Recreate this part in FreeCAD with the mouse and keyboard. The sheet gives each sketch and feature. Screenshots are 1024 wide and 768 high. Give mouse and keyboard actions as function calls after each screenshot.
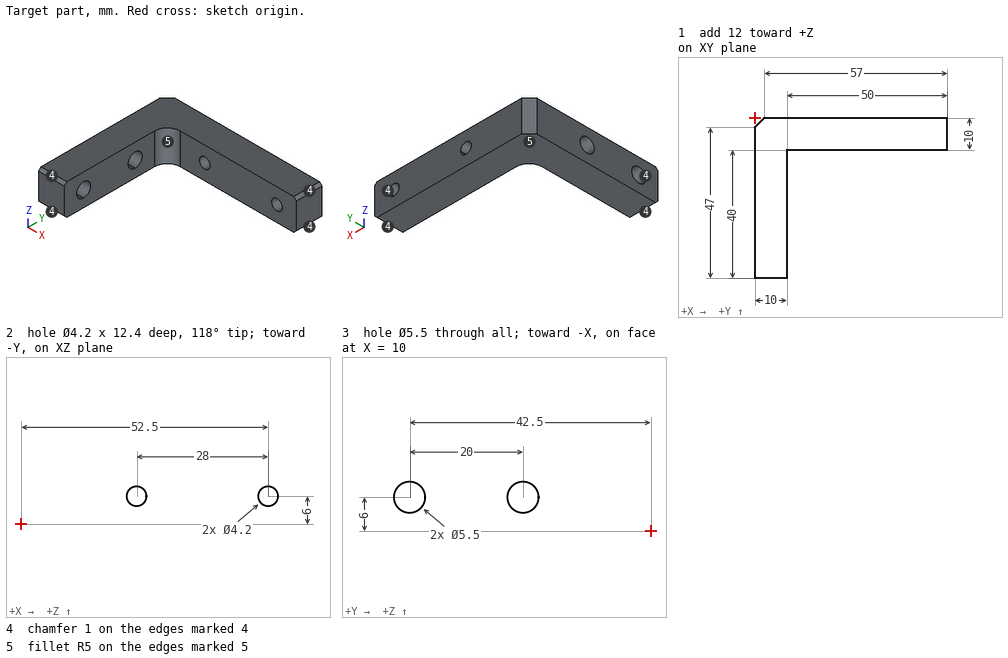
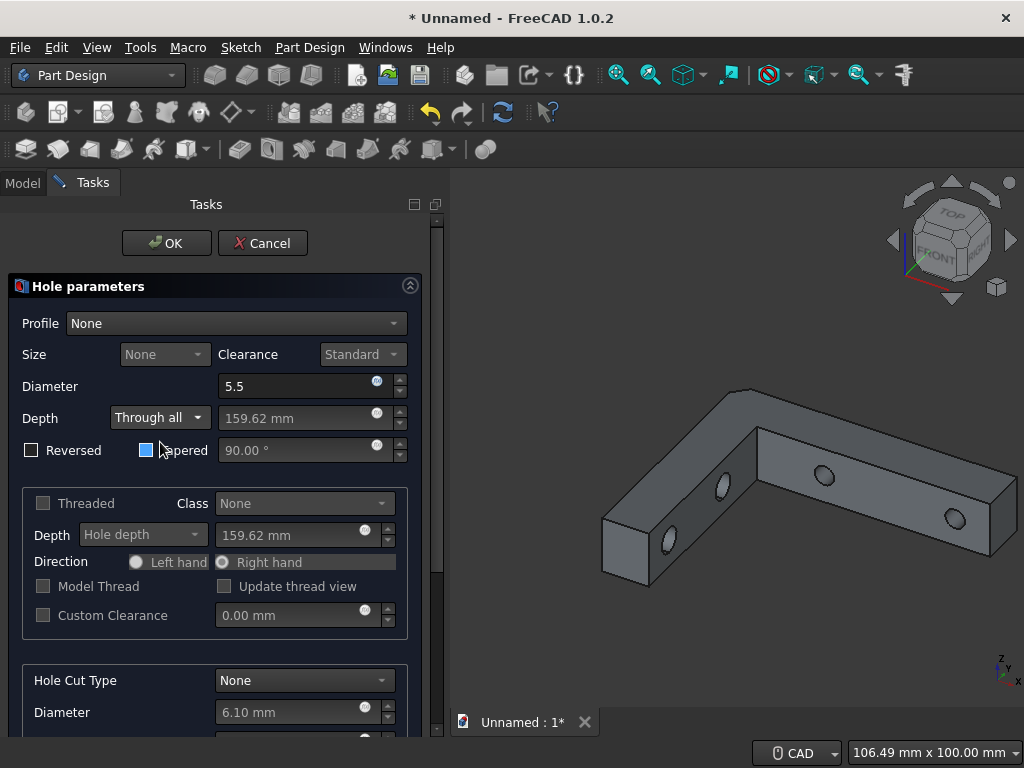
click(167, 243)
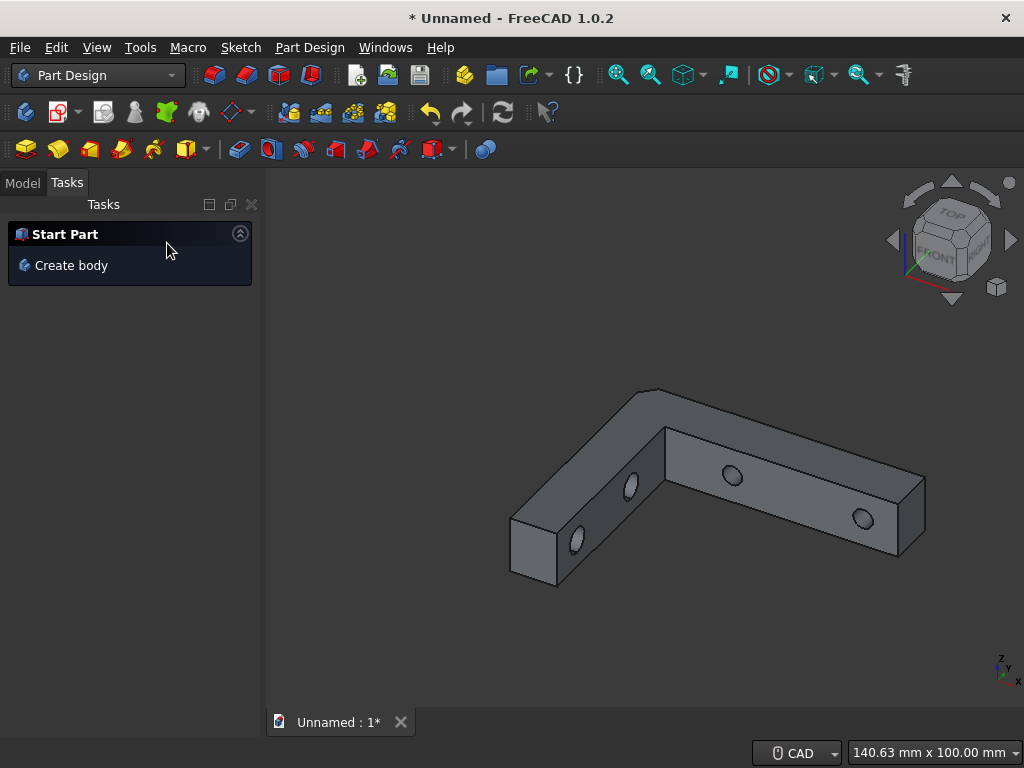
click(534, 525)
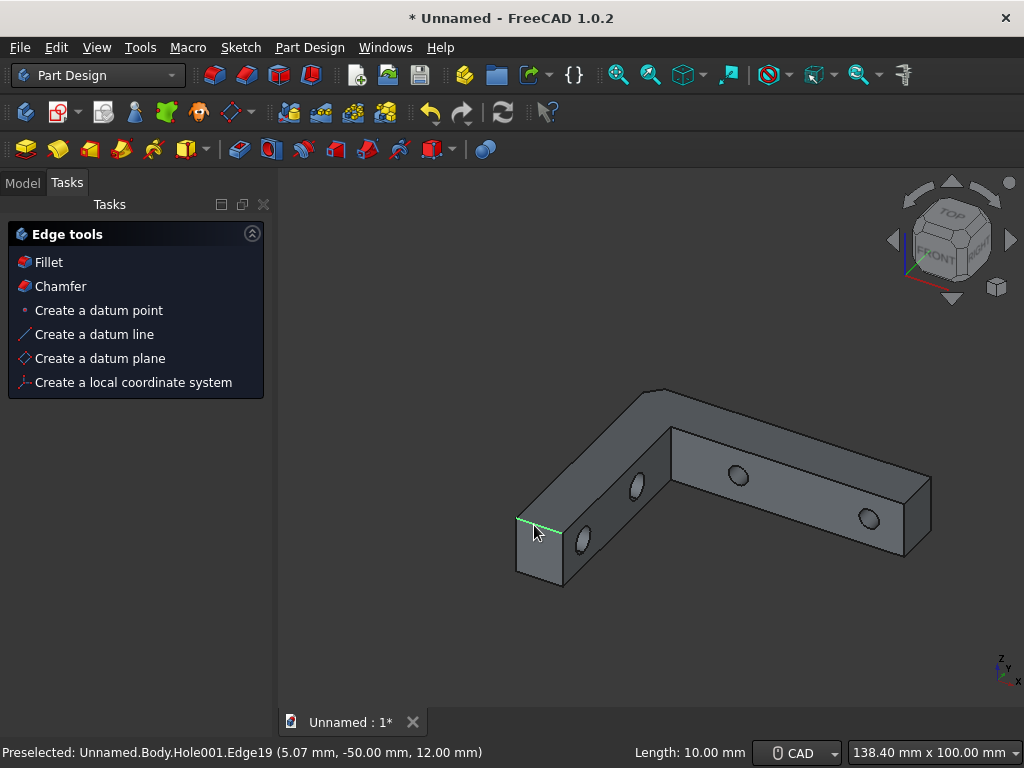
click(918, 490, ctrl)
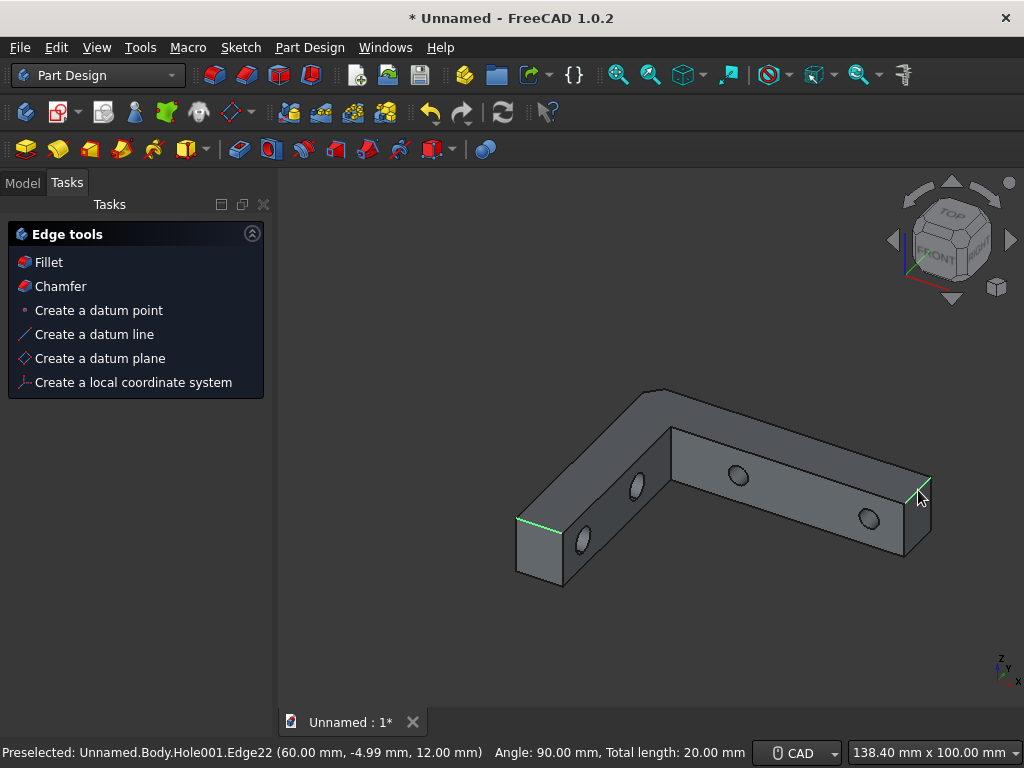
key(0)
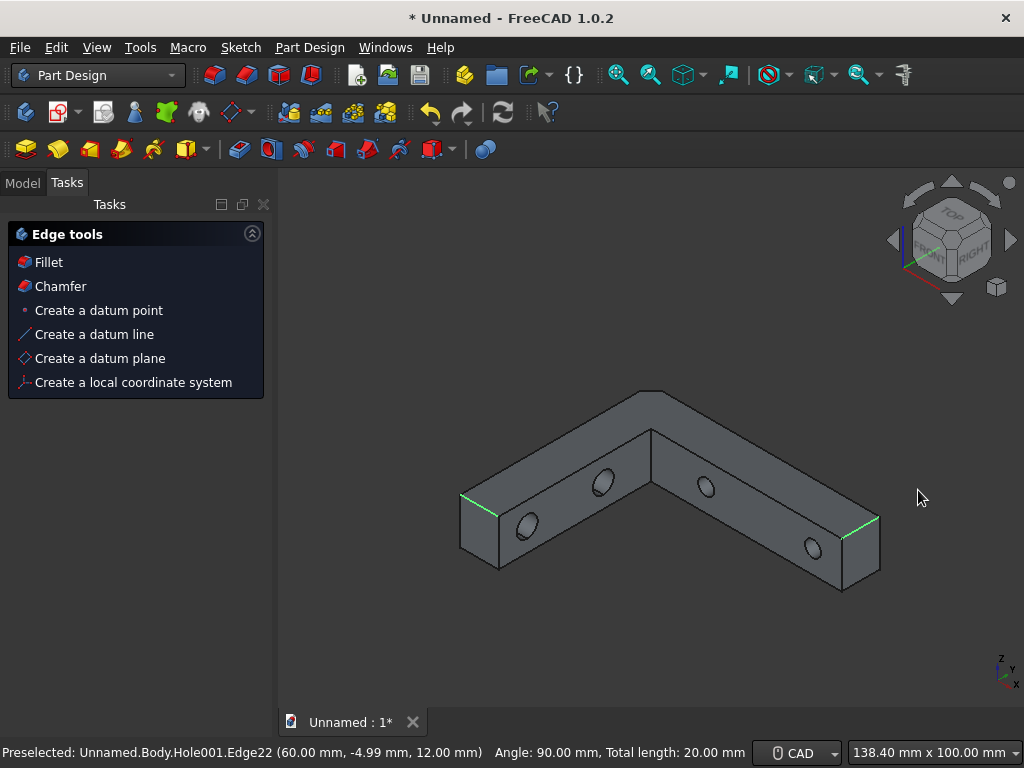
key(2)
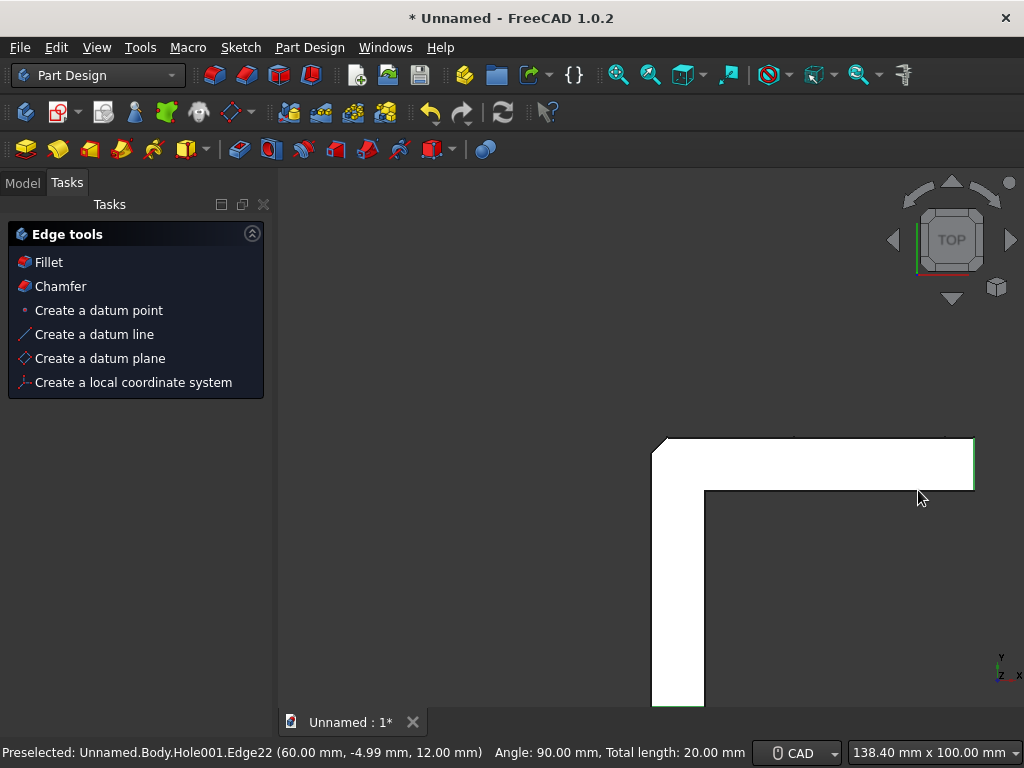
key(1)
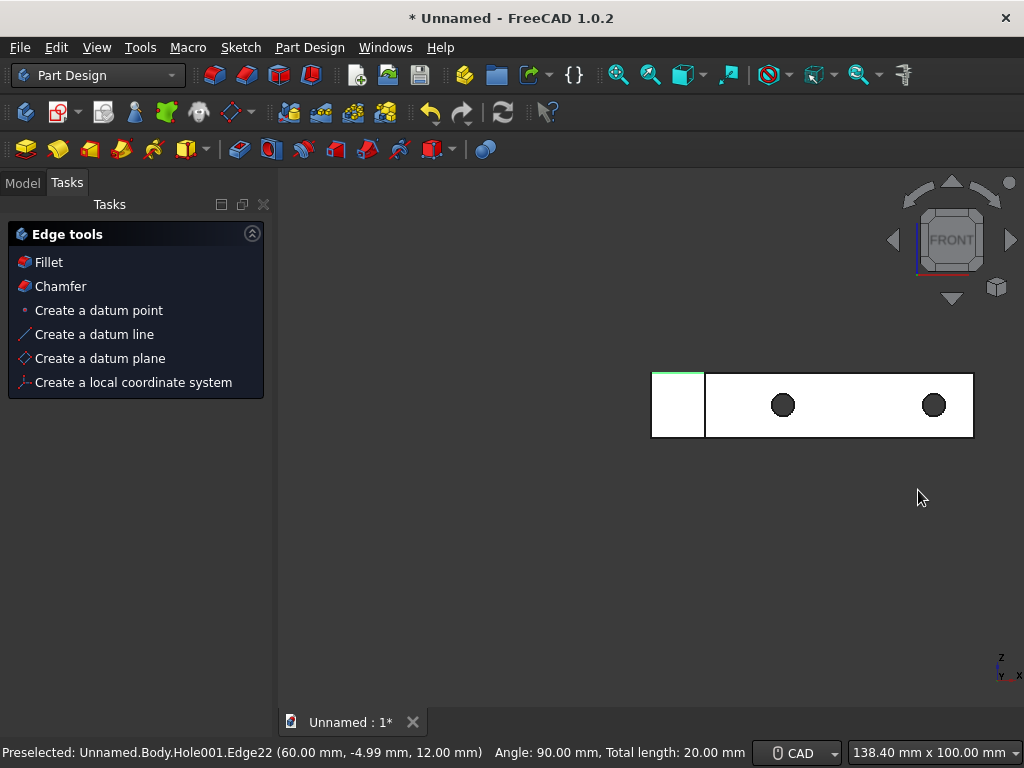
key(v)
key(f)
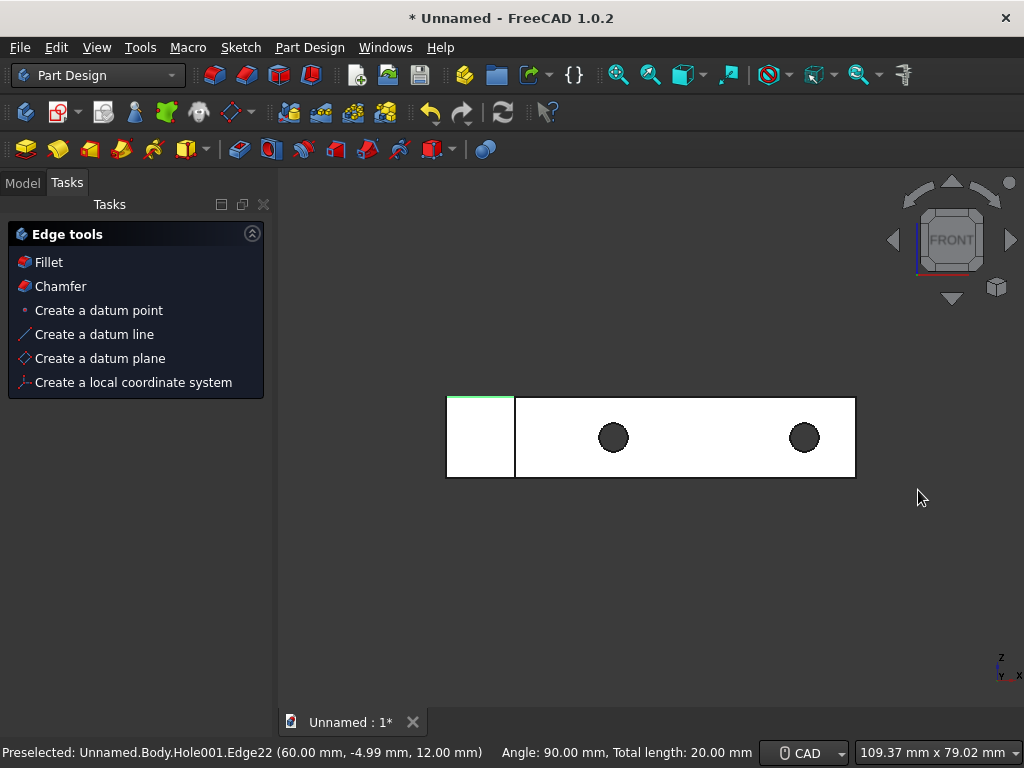
click(480, 477, ctrl)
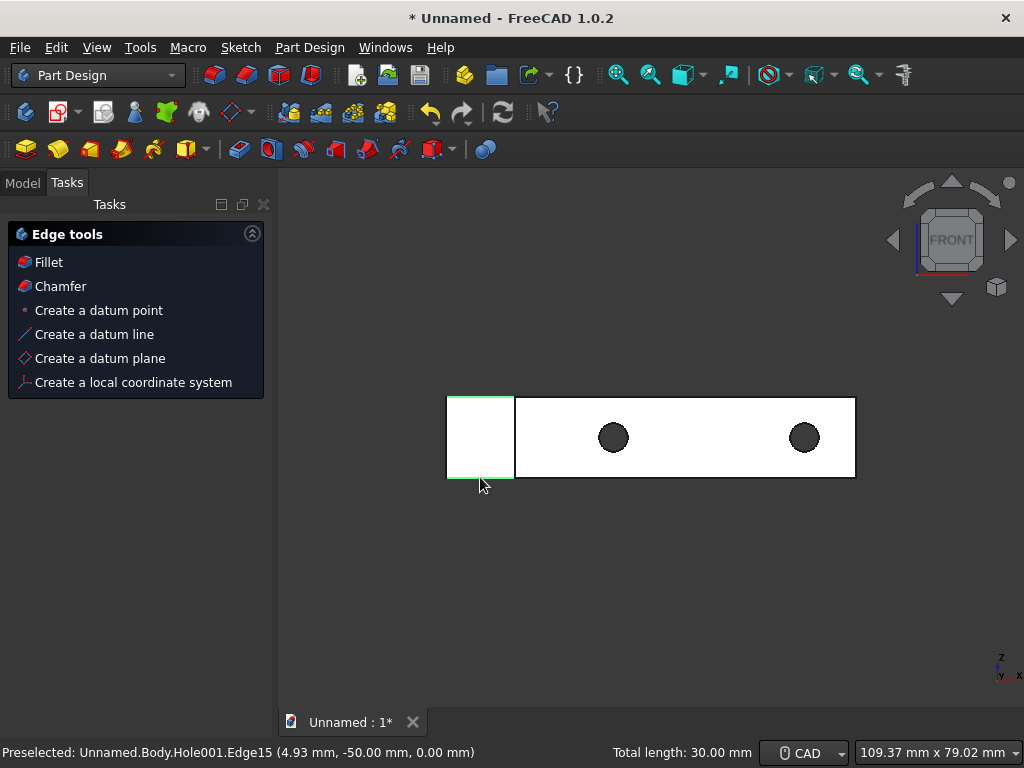
key(3)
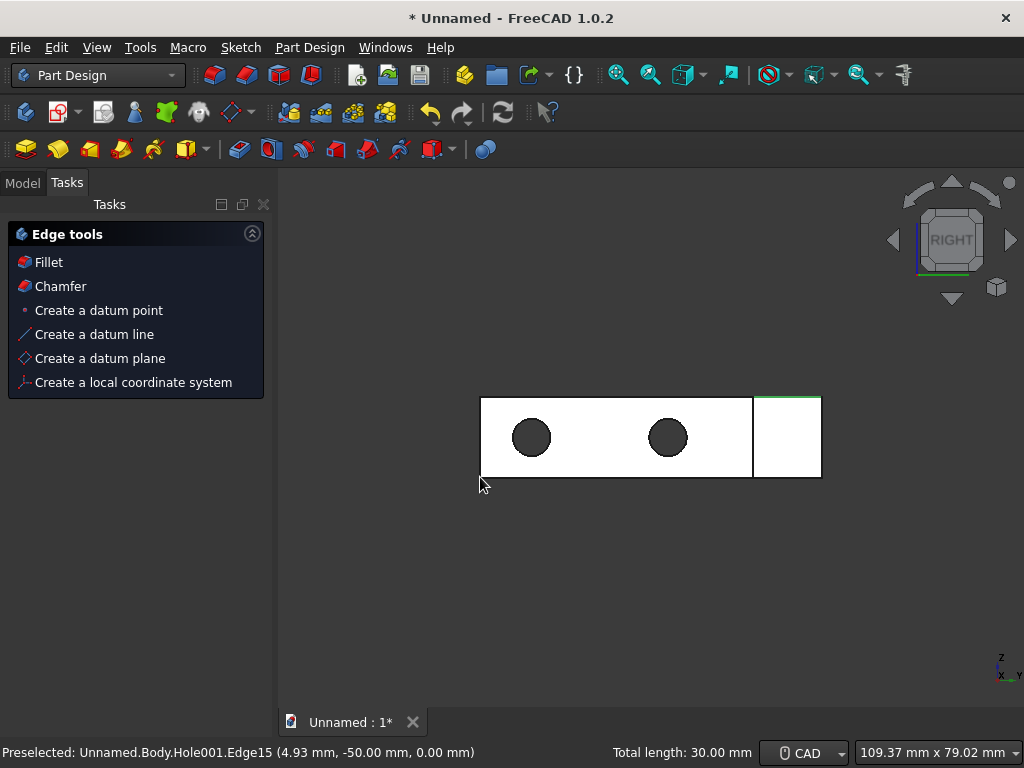
click(787, 477, ctrl)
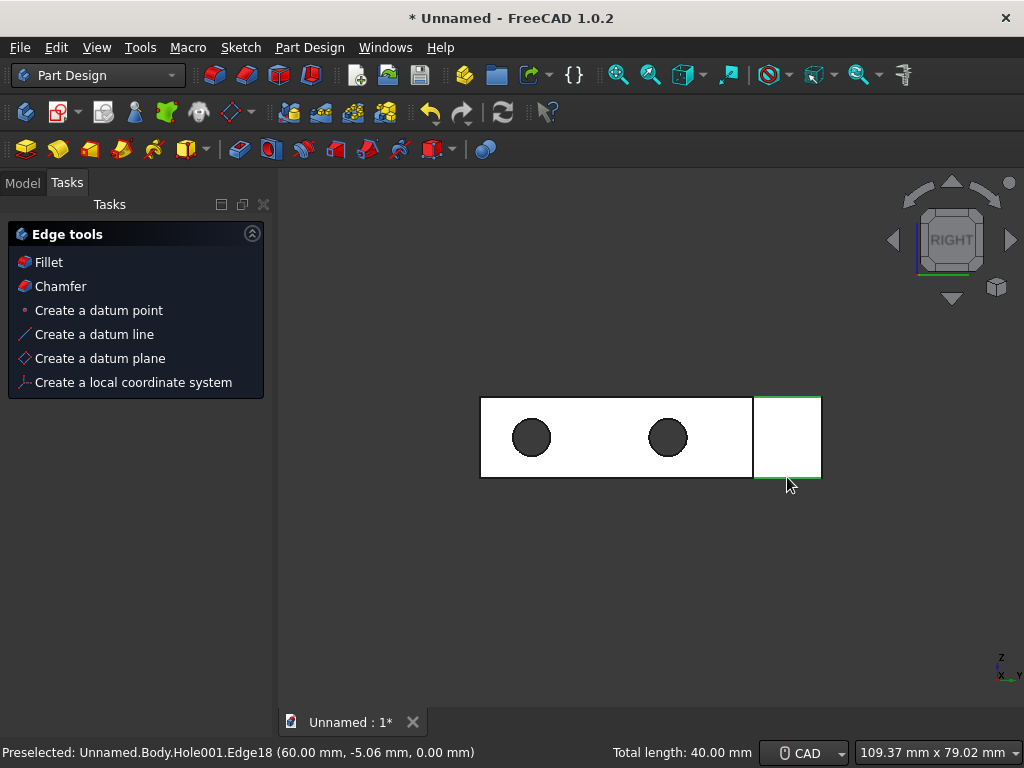
click(248, 76)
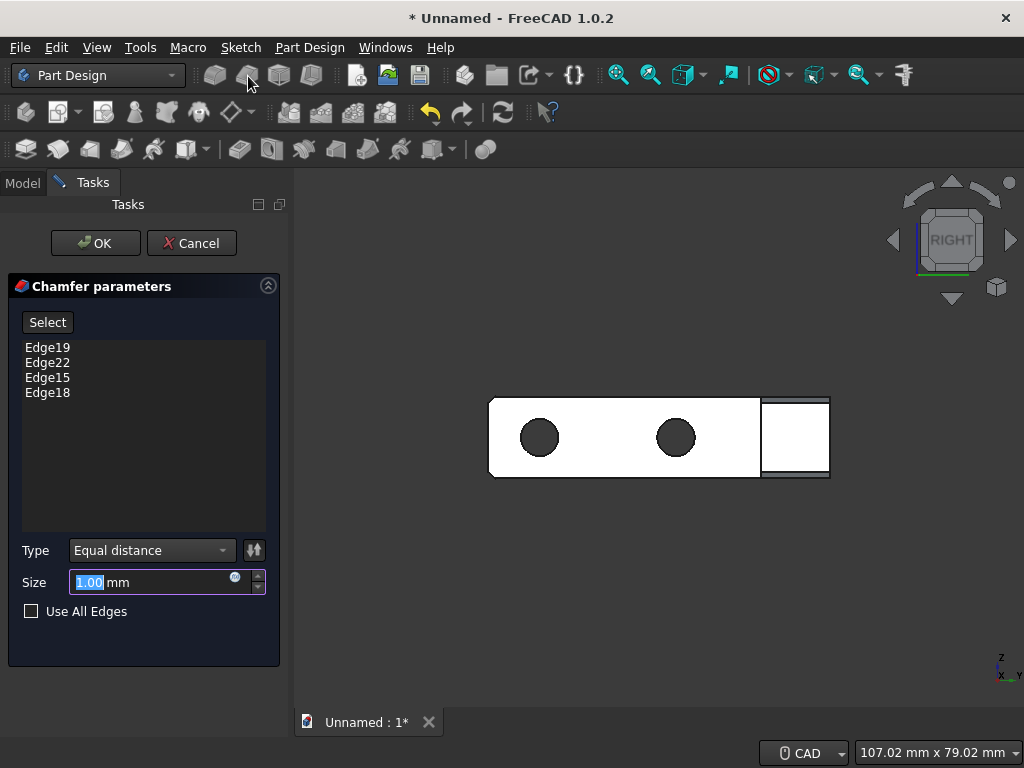
text(1)
key(Tab)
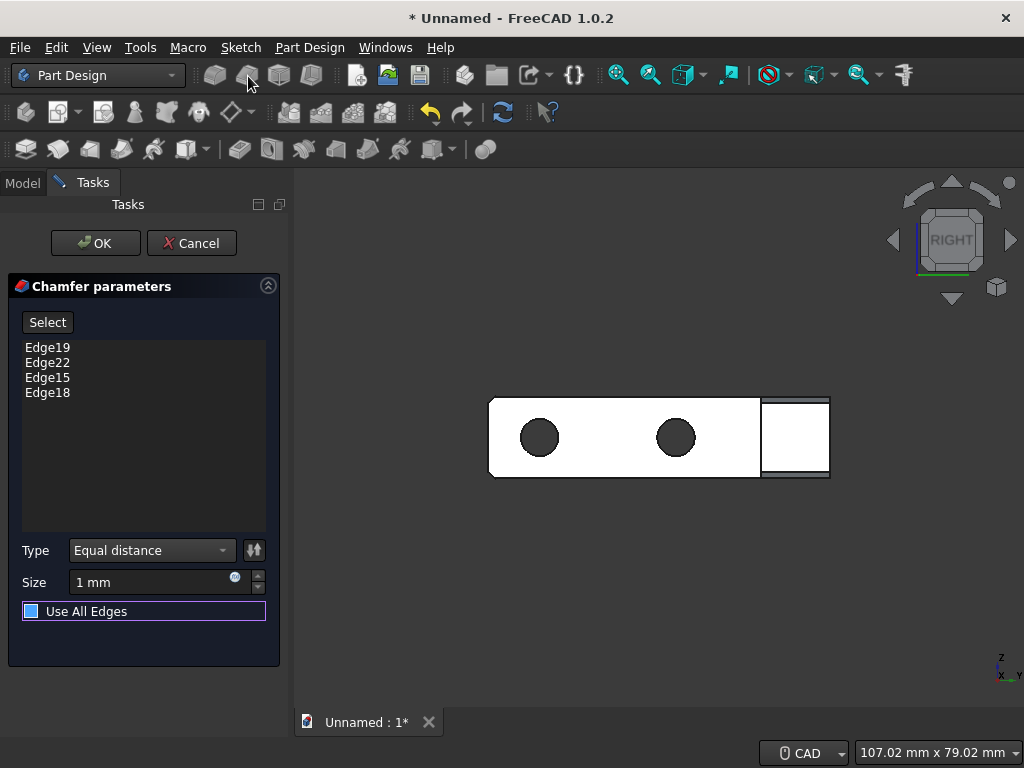
click(96, 243)